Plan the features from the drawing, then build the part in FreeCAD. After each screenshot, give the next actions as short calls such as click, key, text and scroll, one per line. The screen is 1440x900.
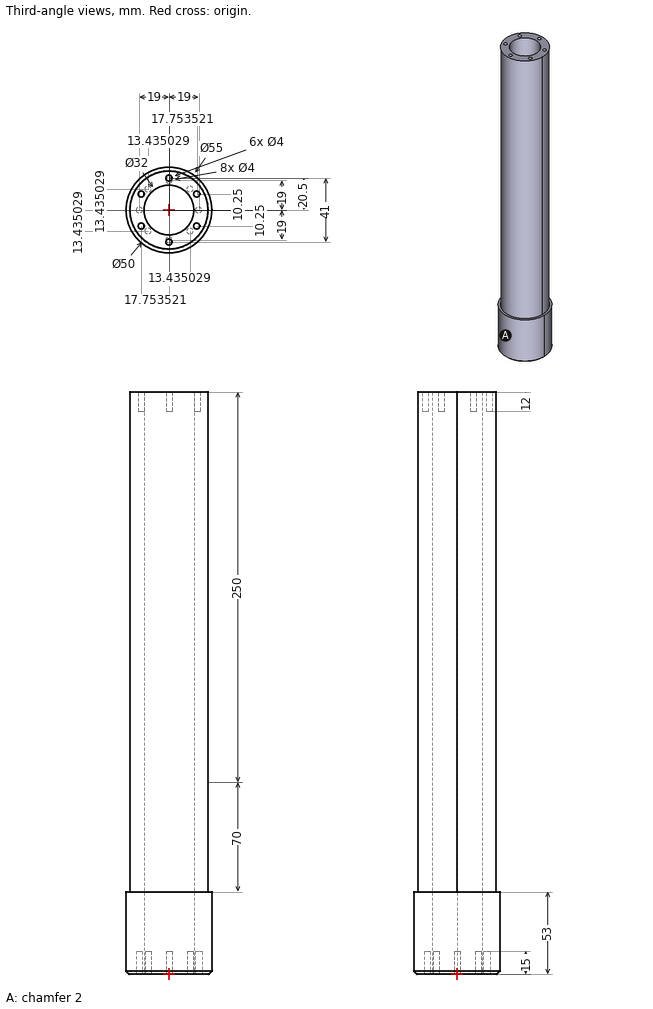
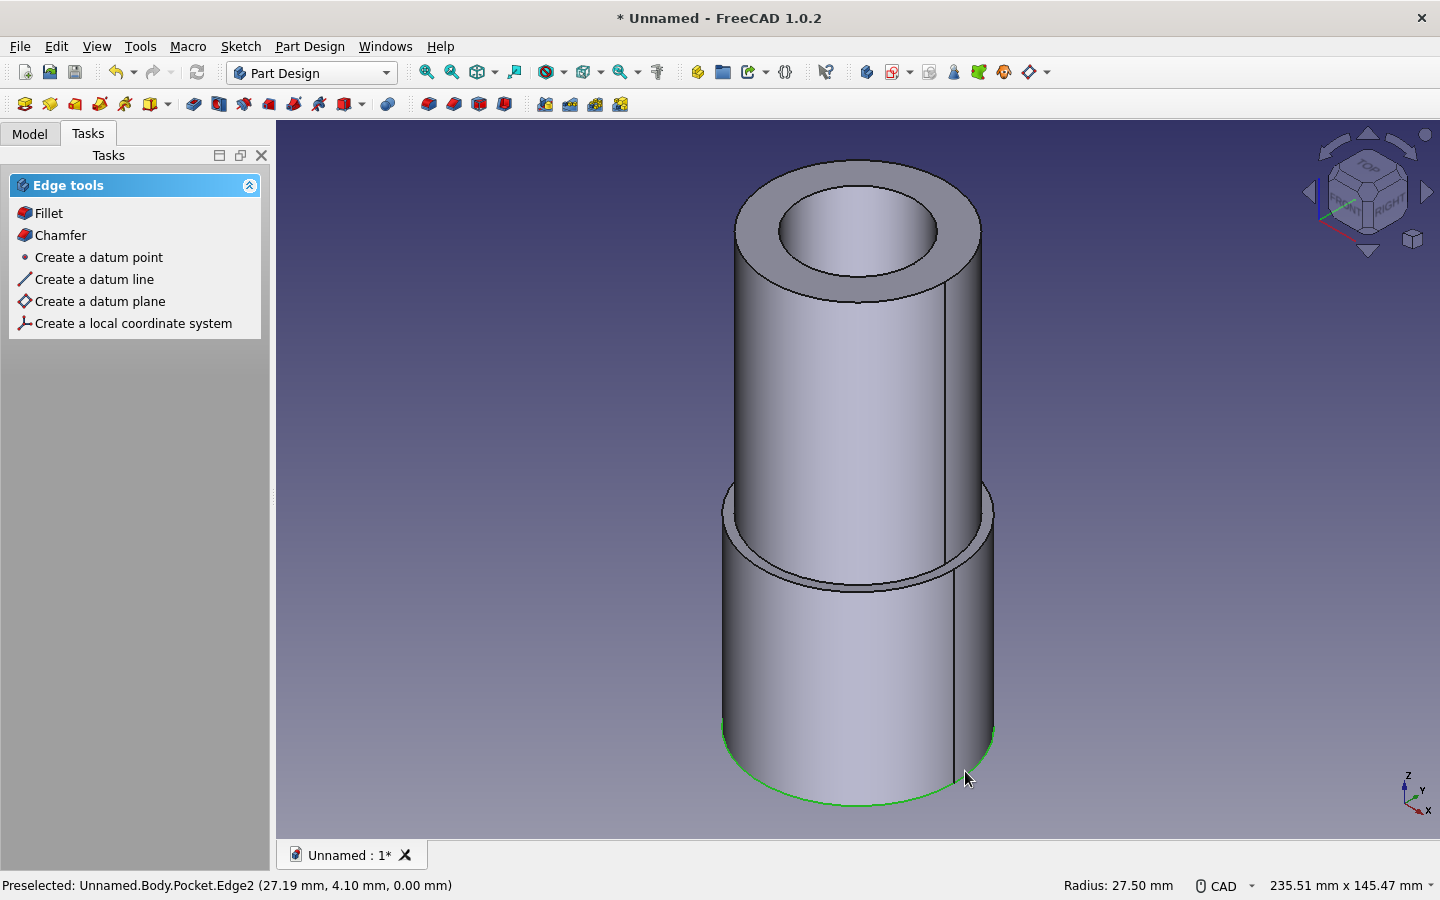
click(454, 104)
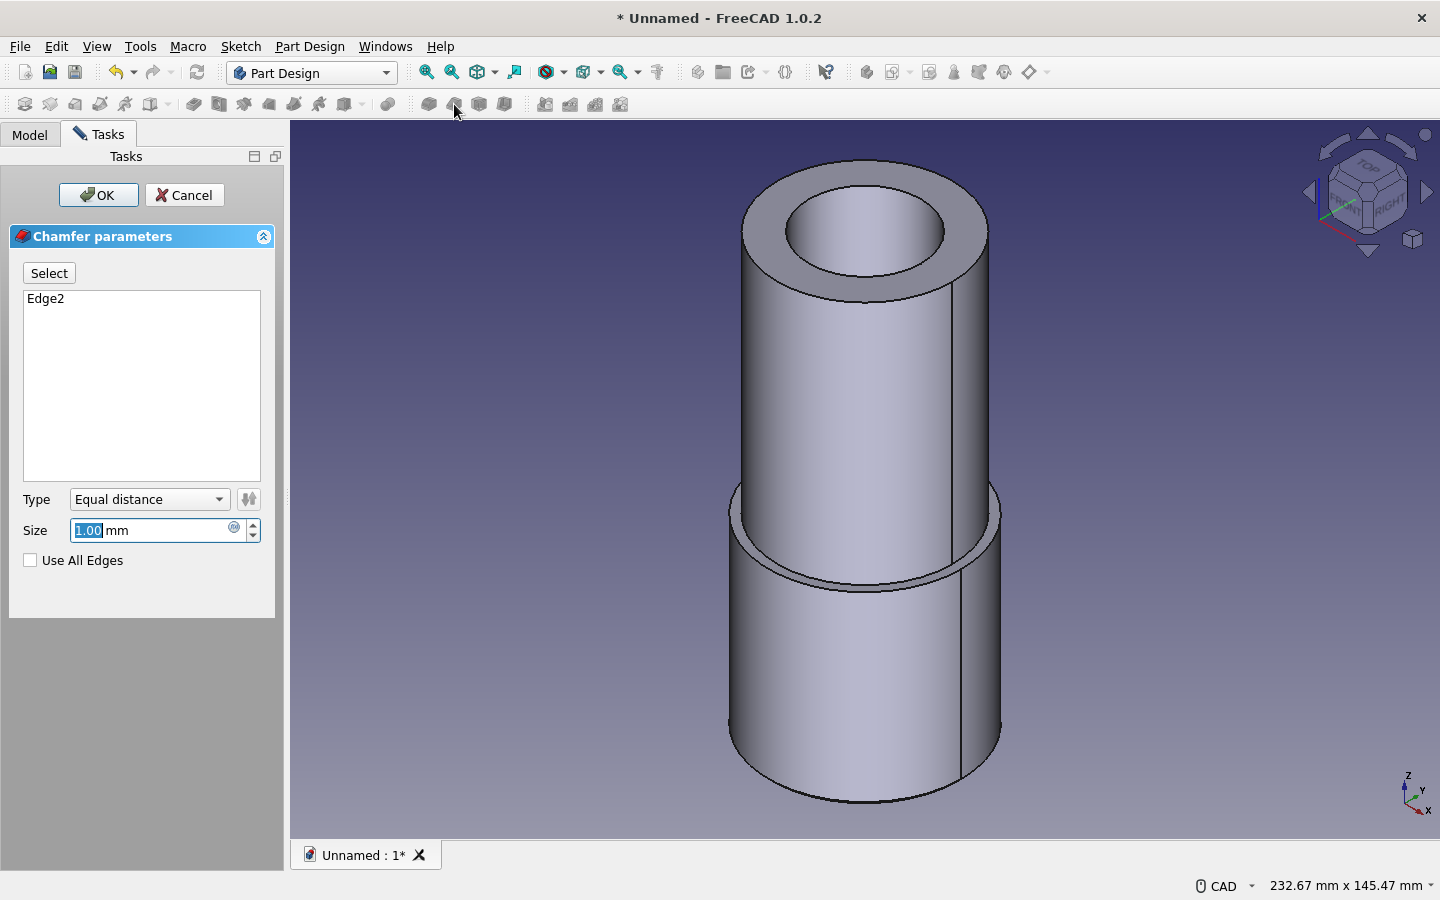
text(2)
key(Tab)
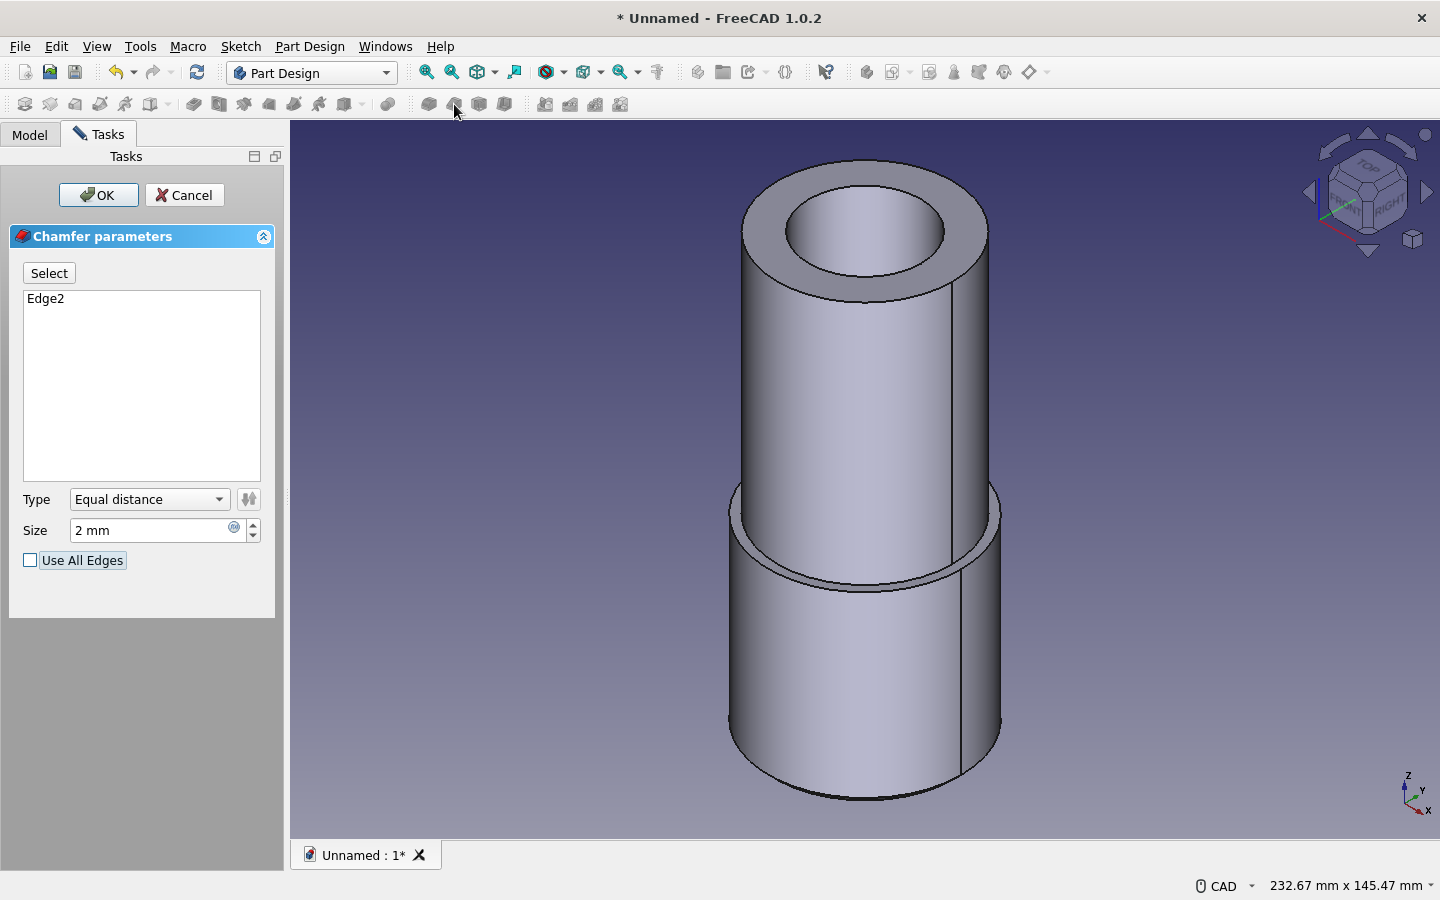
click(99, 195)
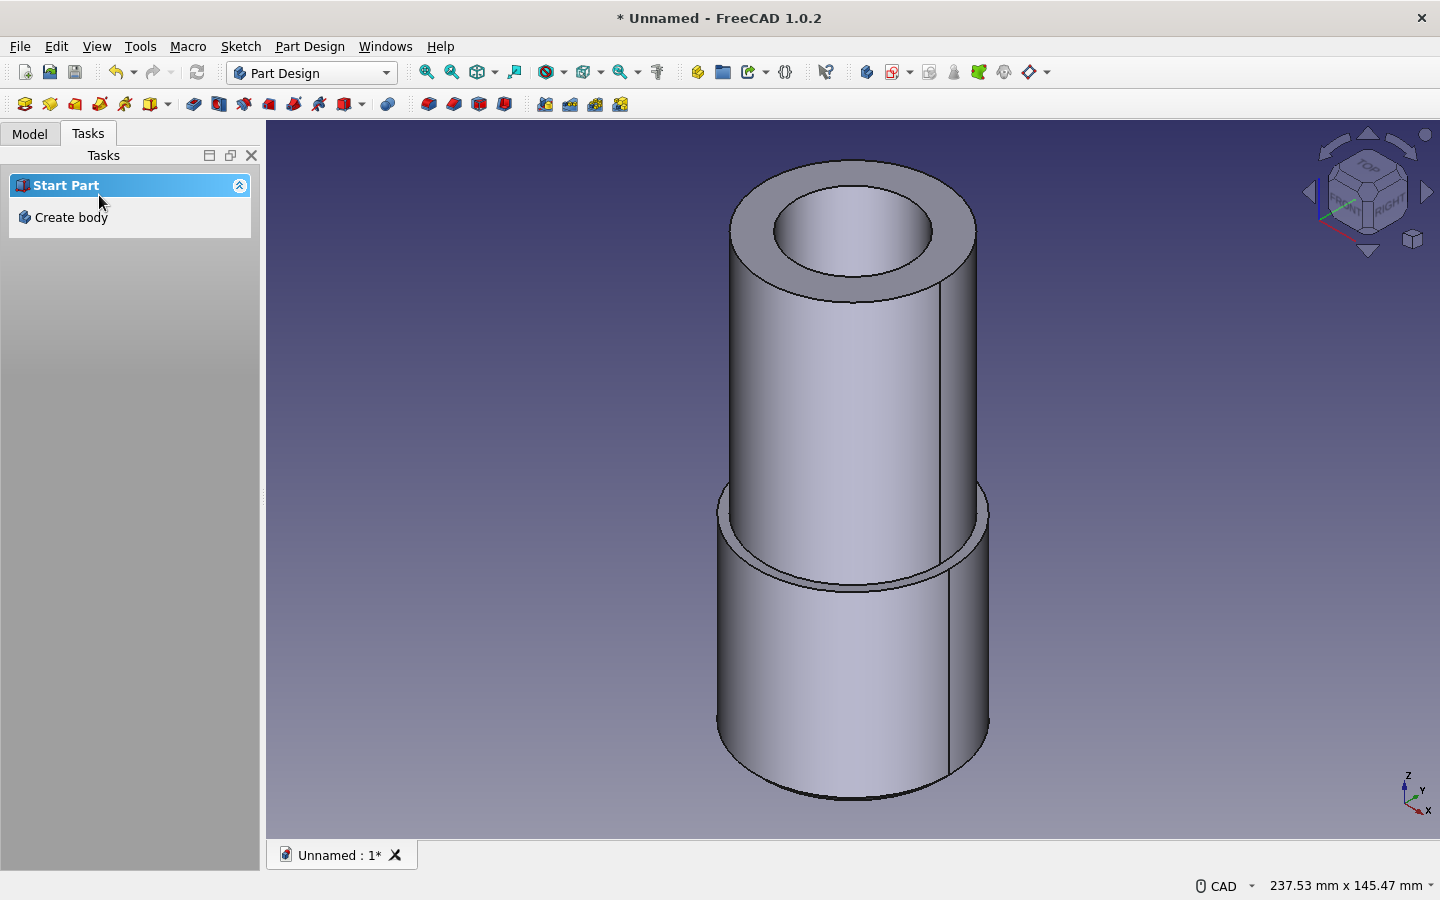
click(427, 72)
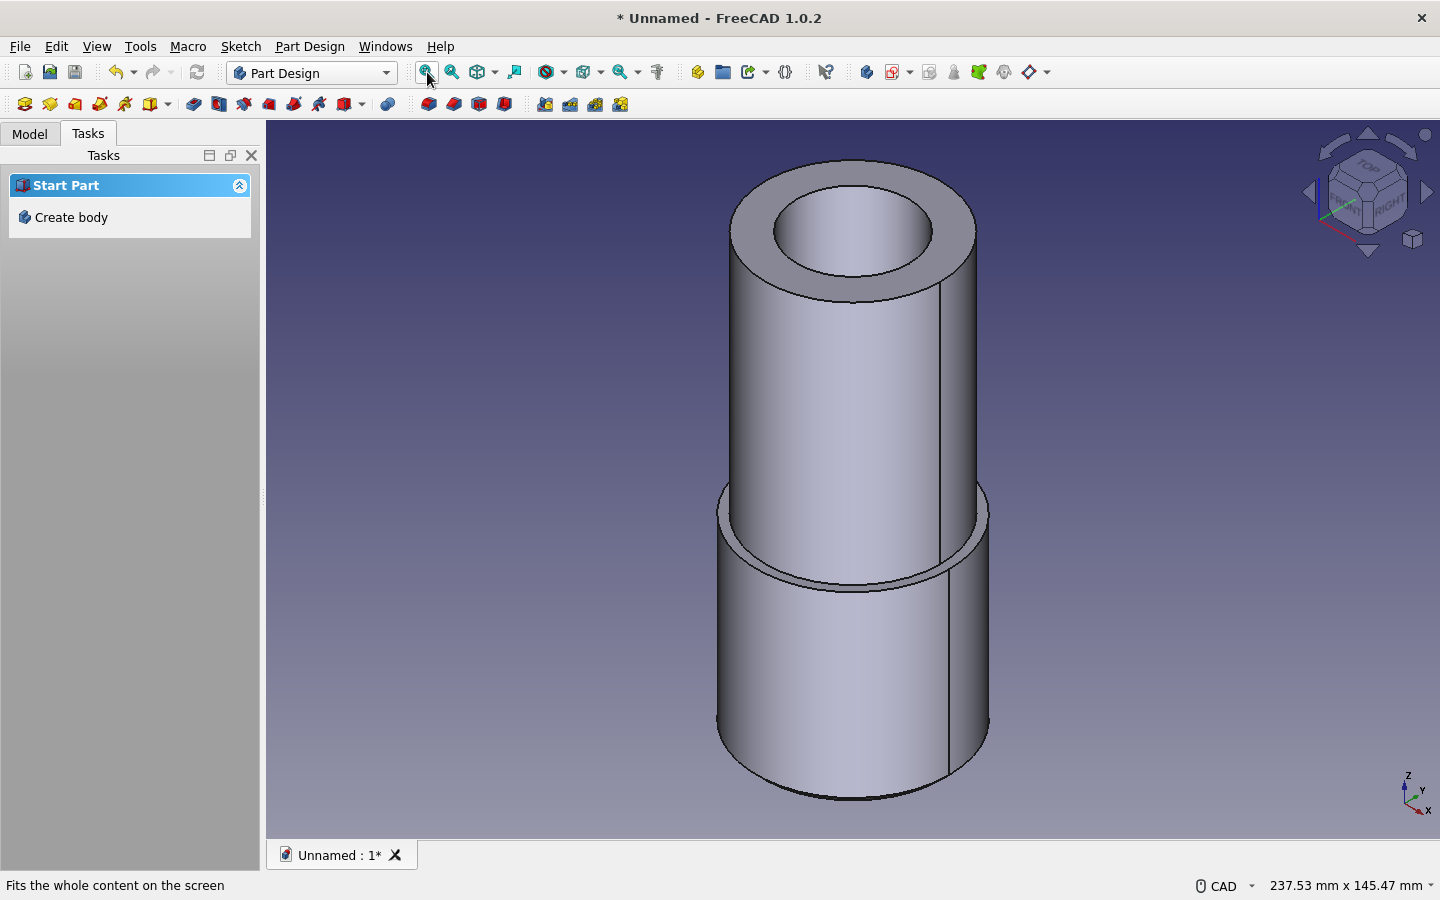
click(853, 173)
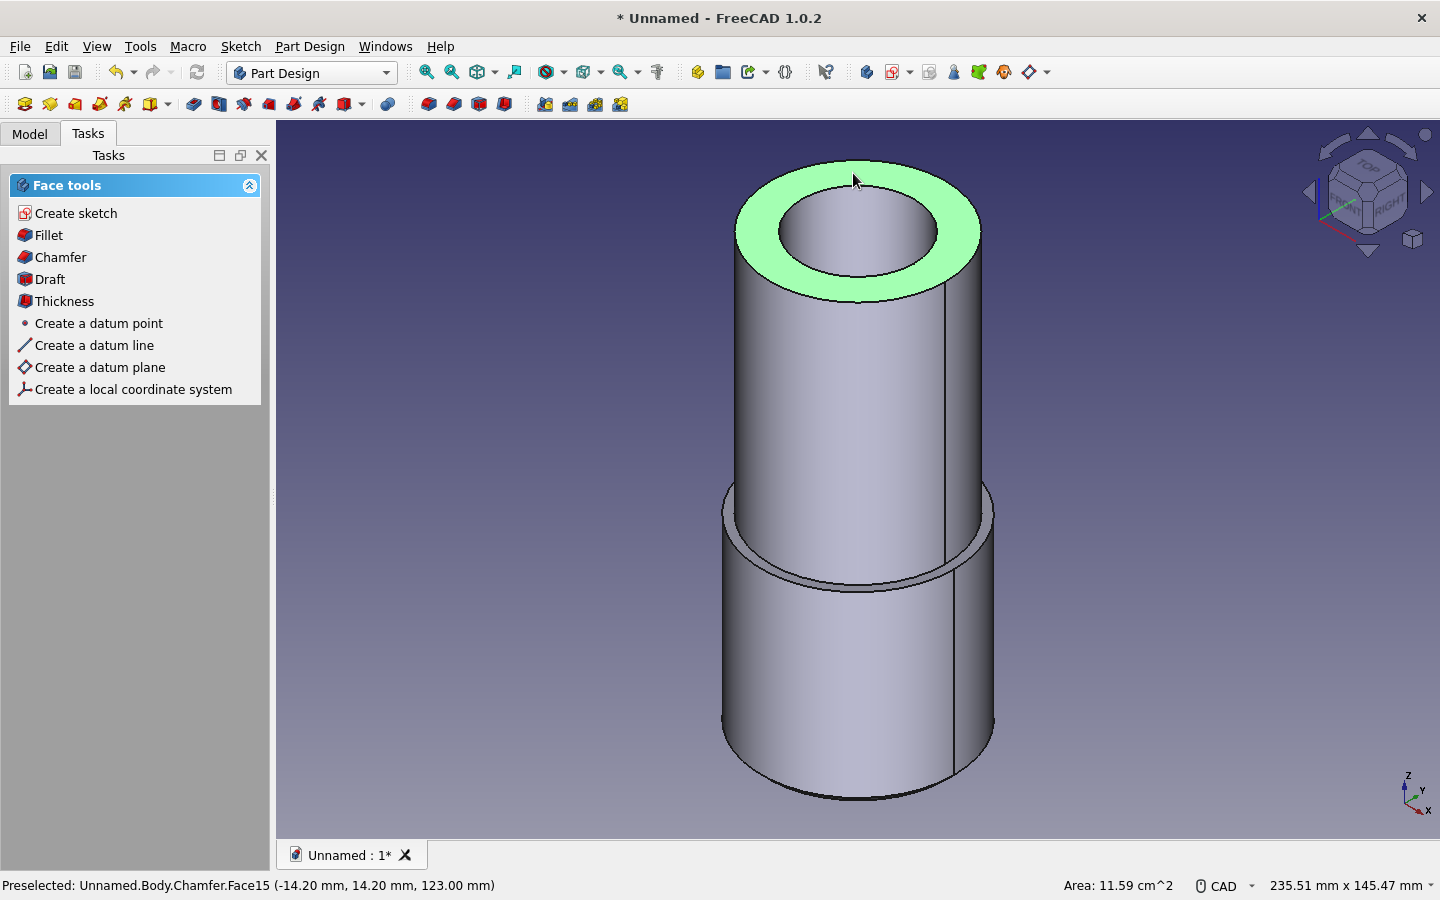
click(892, 72)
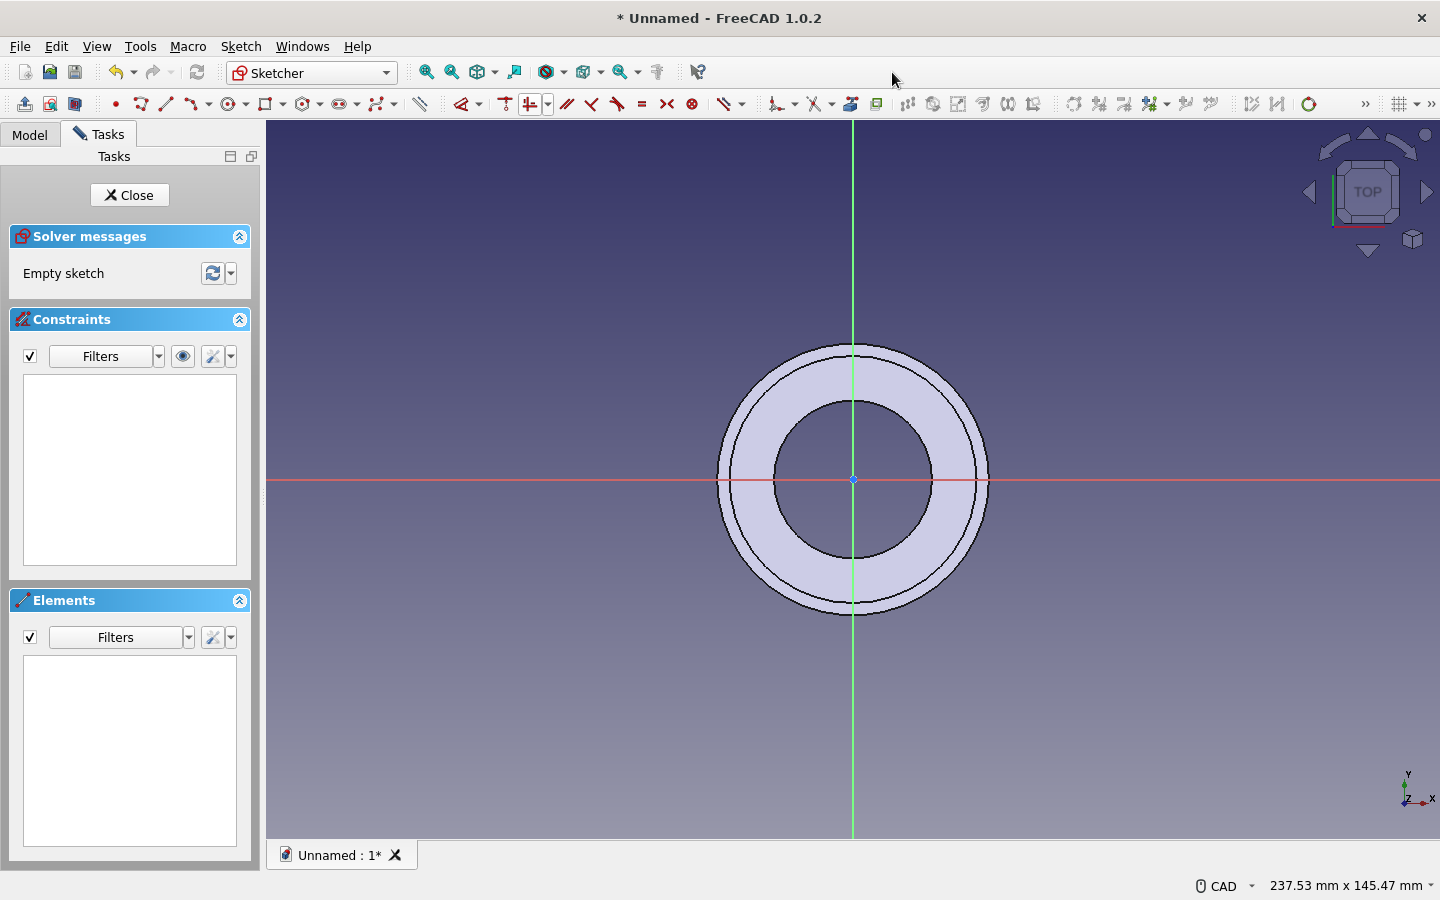
scroll(936, 480, up, 3)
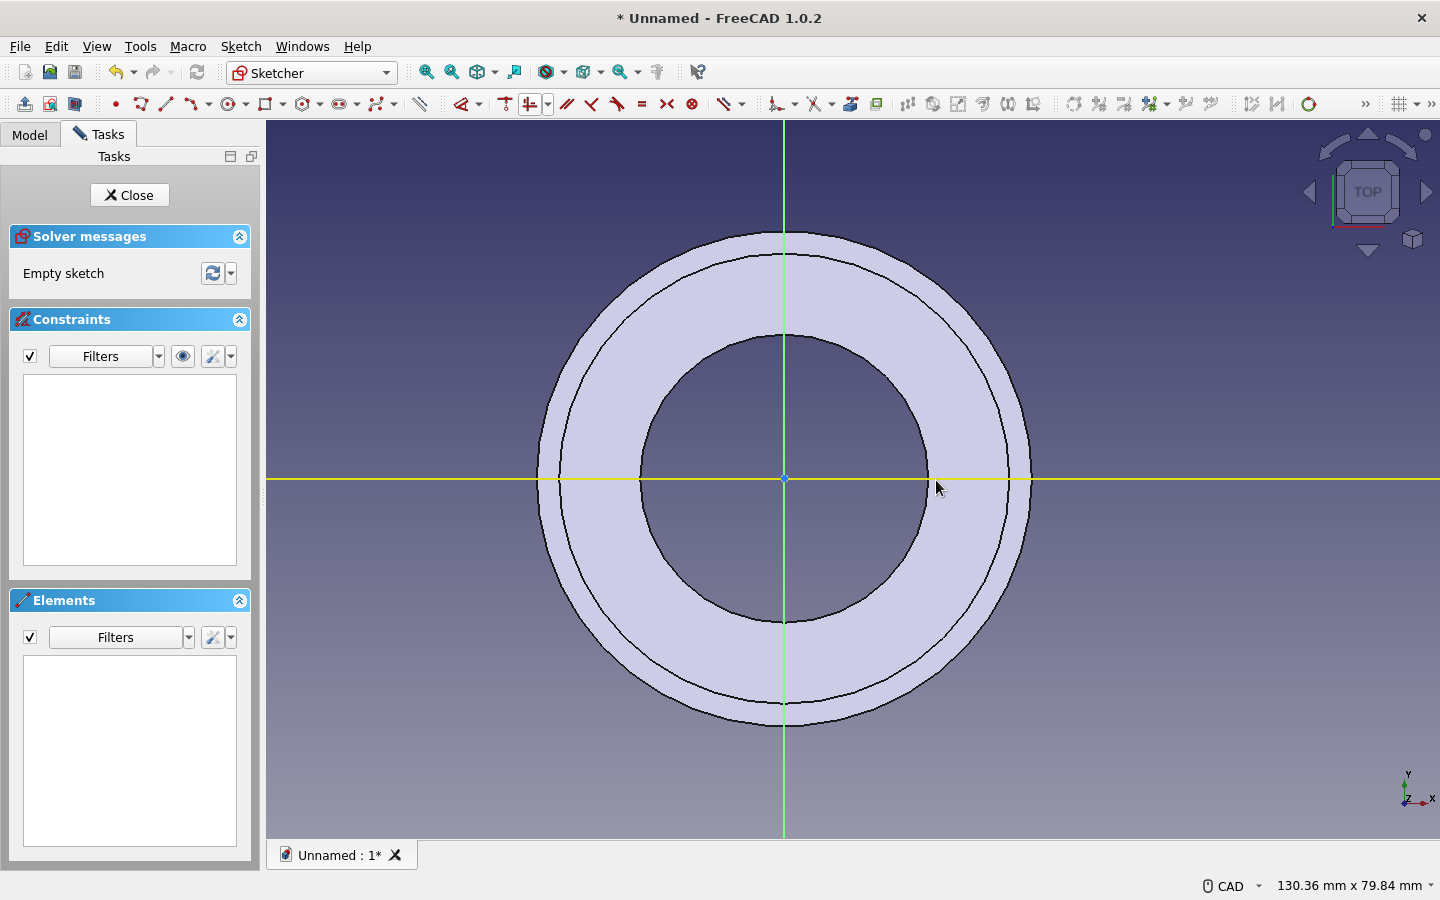
click(228, 104)